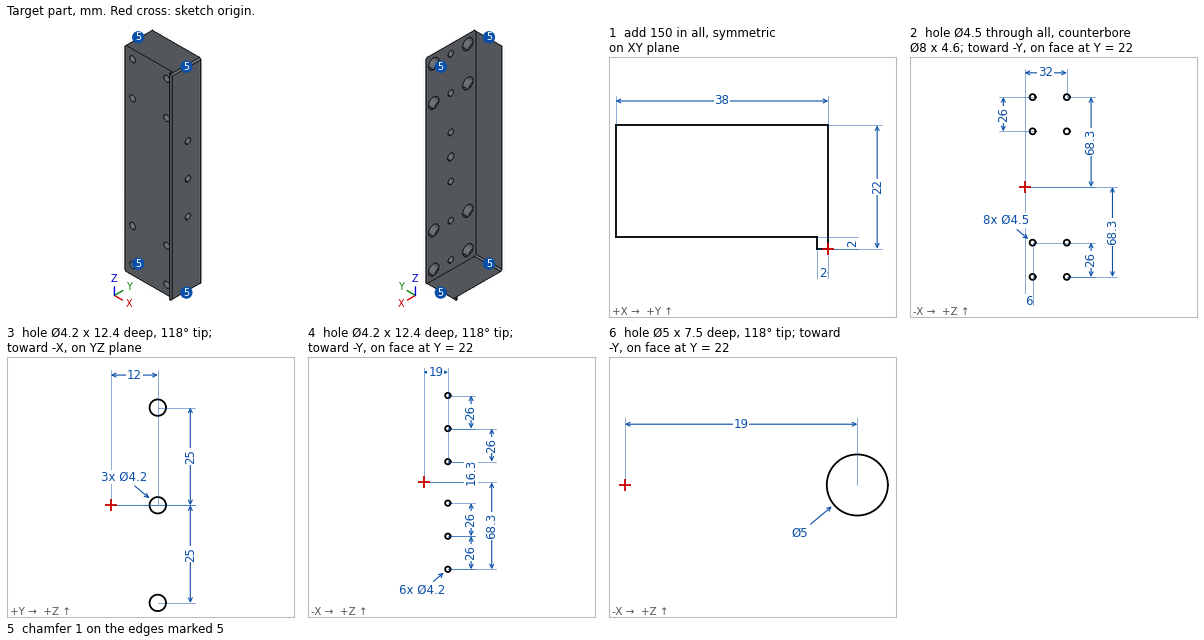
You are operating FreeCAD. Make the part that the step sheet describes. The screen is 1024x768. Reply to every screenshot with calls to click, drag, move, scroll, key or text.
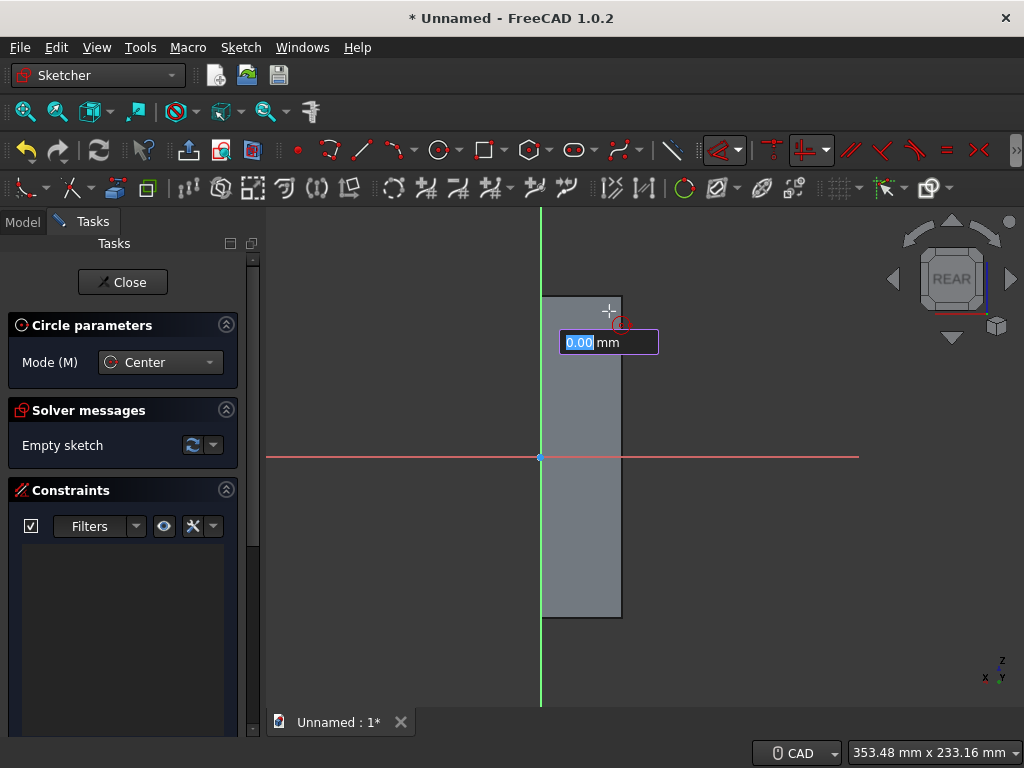
scroll(613, 307, up, 6)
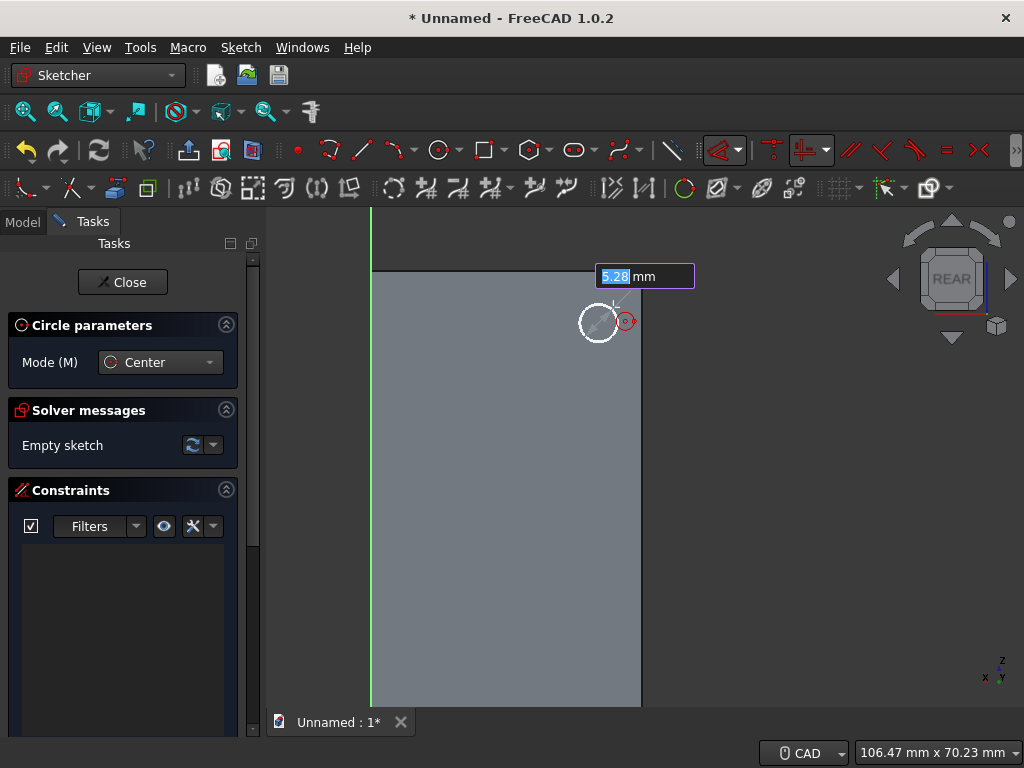
click(610, 307)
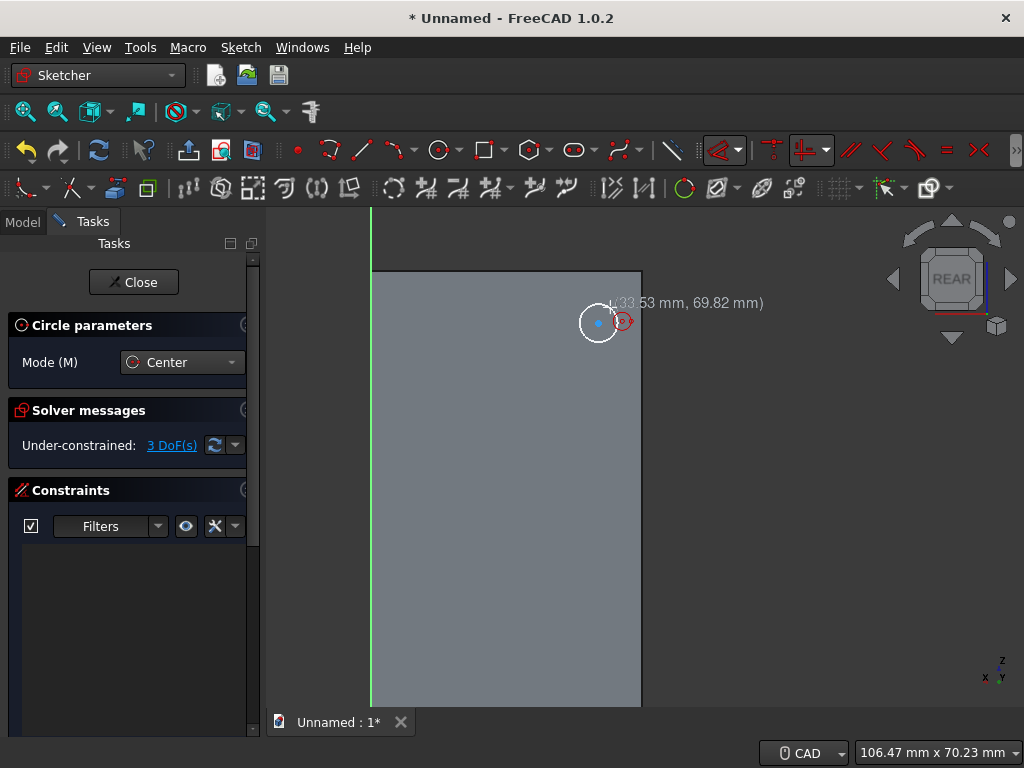
scroll(612, 307, down, 6)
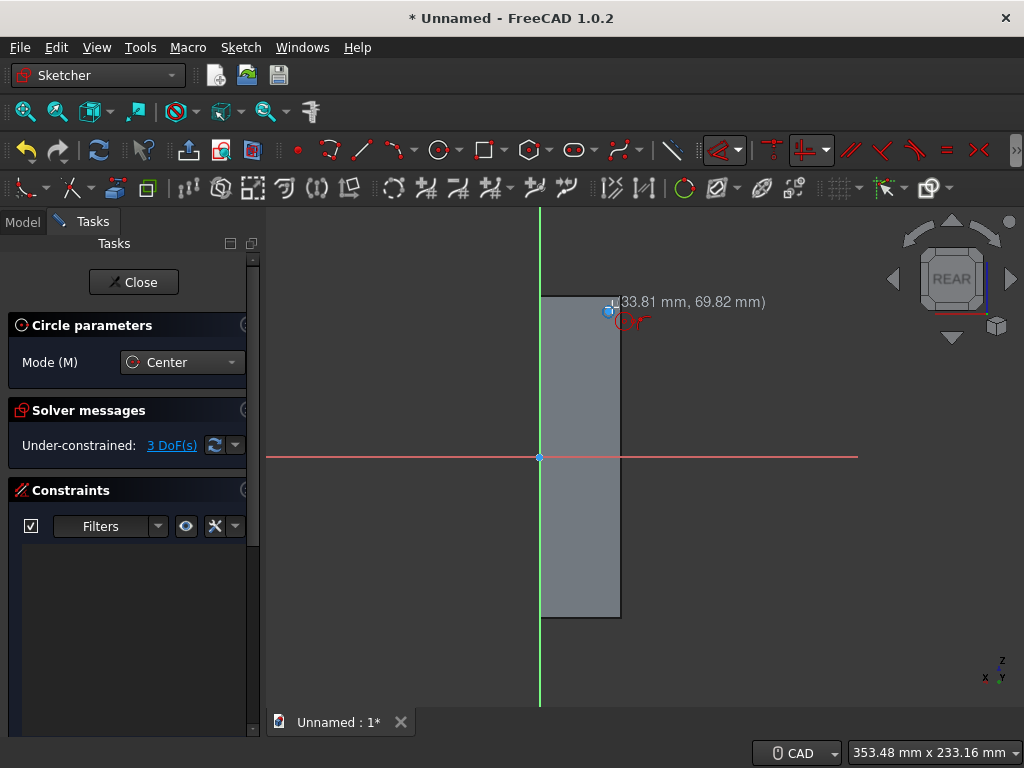
scroll(608, 604, up, 8)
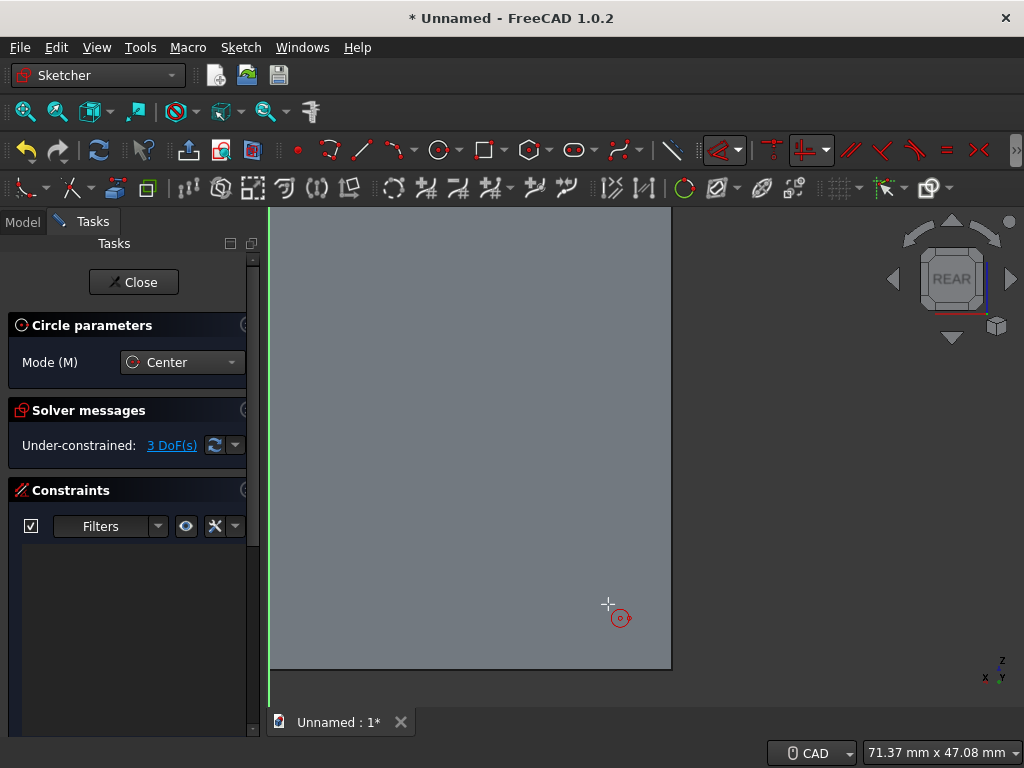
scroll(608, 605, down, 8)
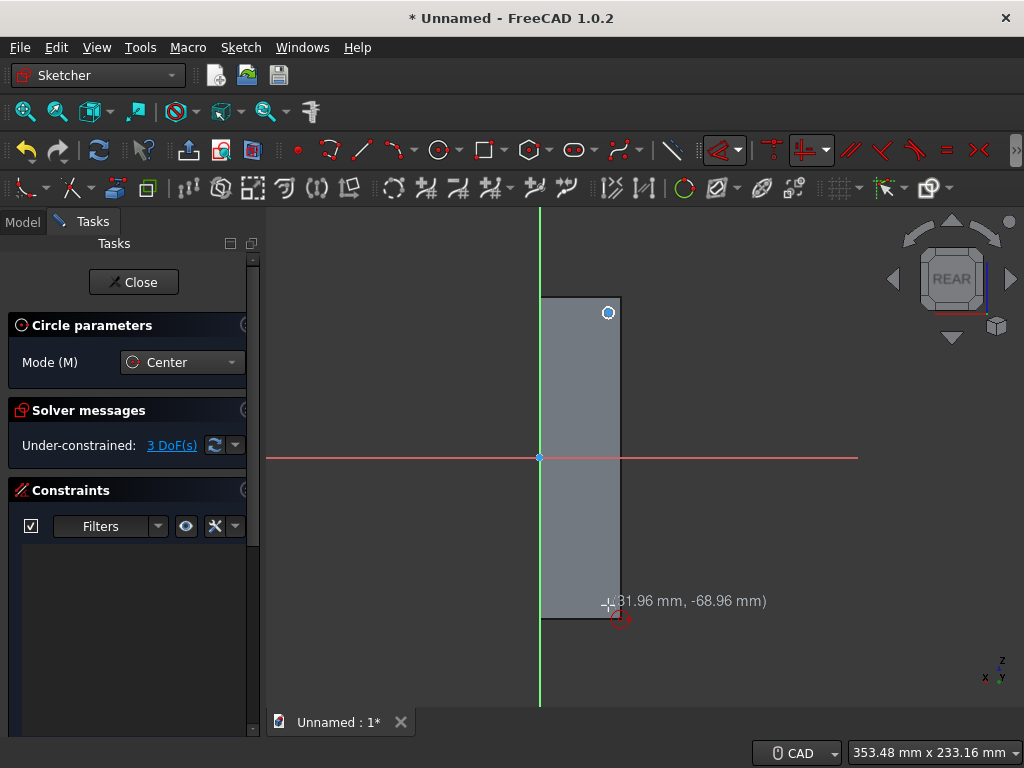
click(608, 604)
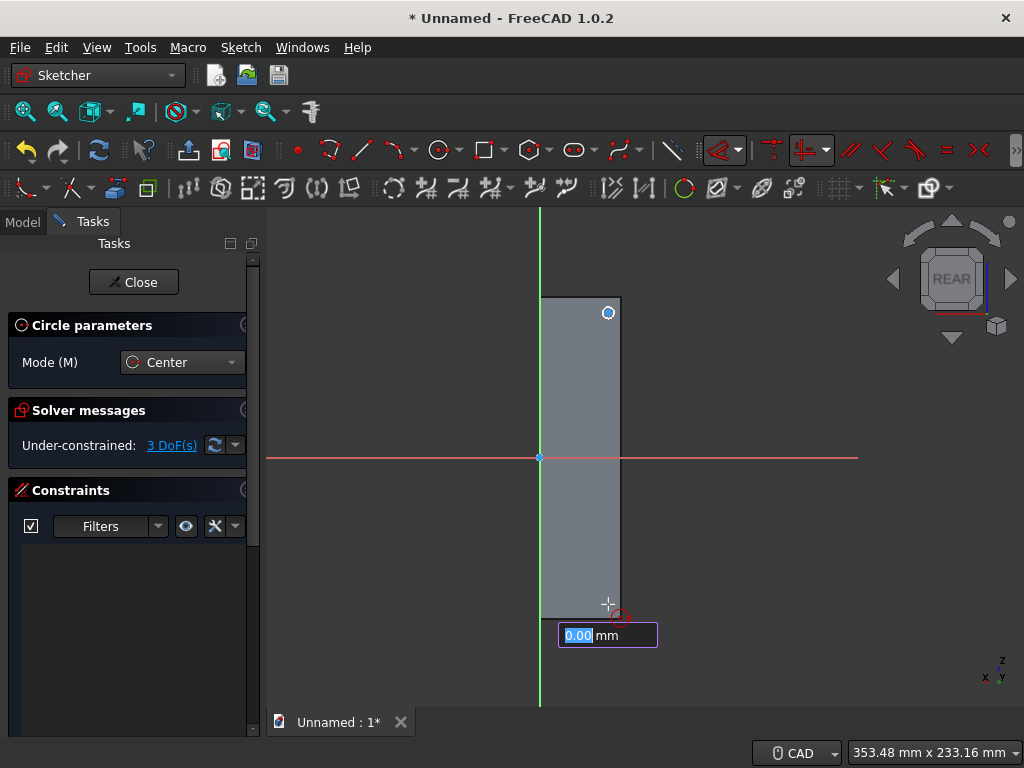
scroll(612, 601, up, 6)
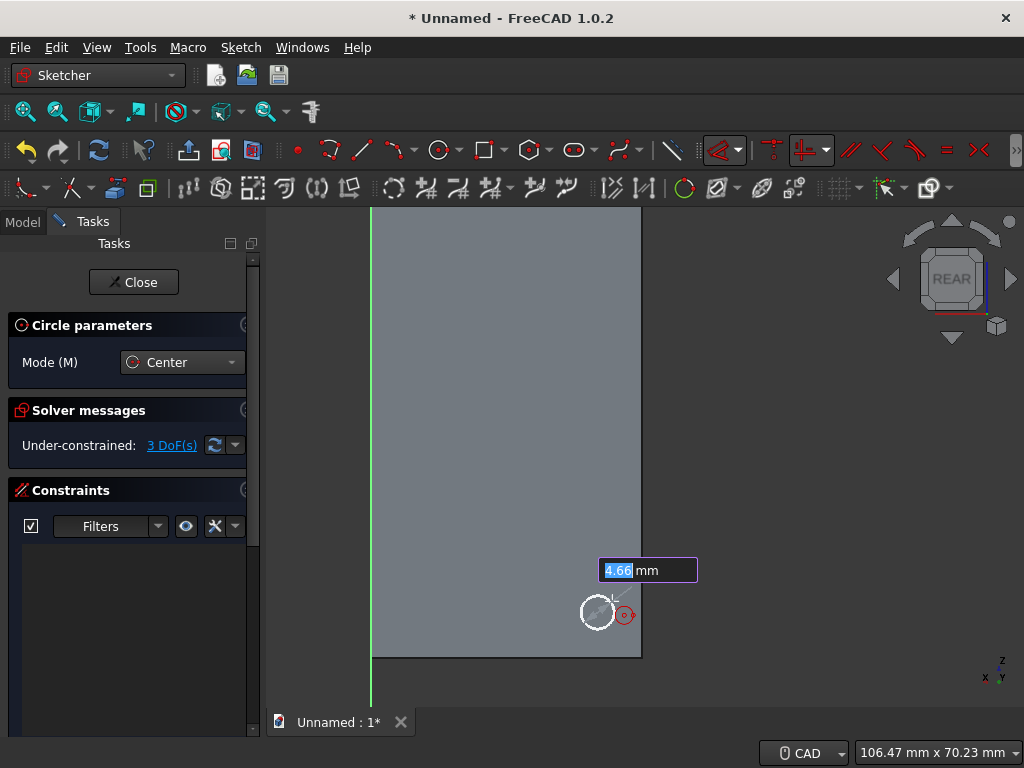
click(610, 599)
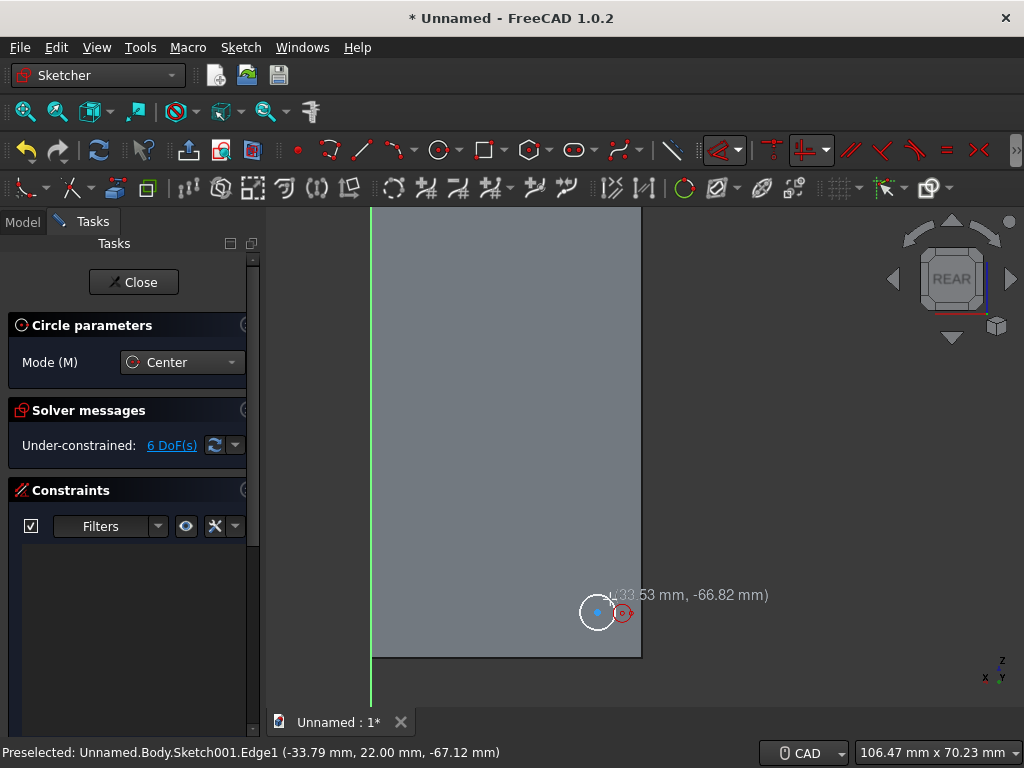
scroll(414, 425, up, 2)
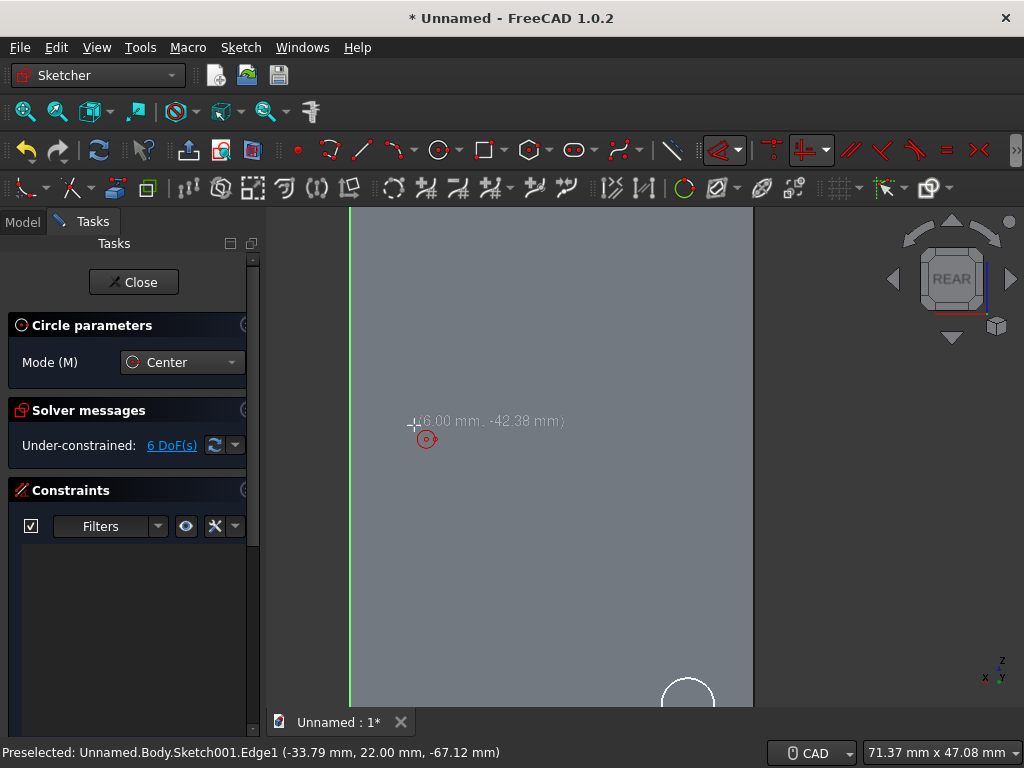
scroll(588, 579, down, 8)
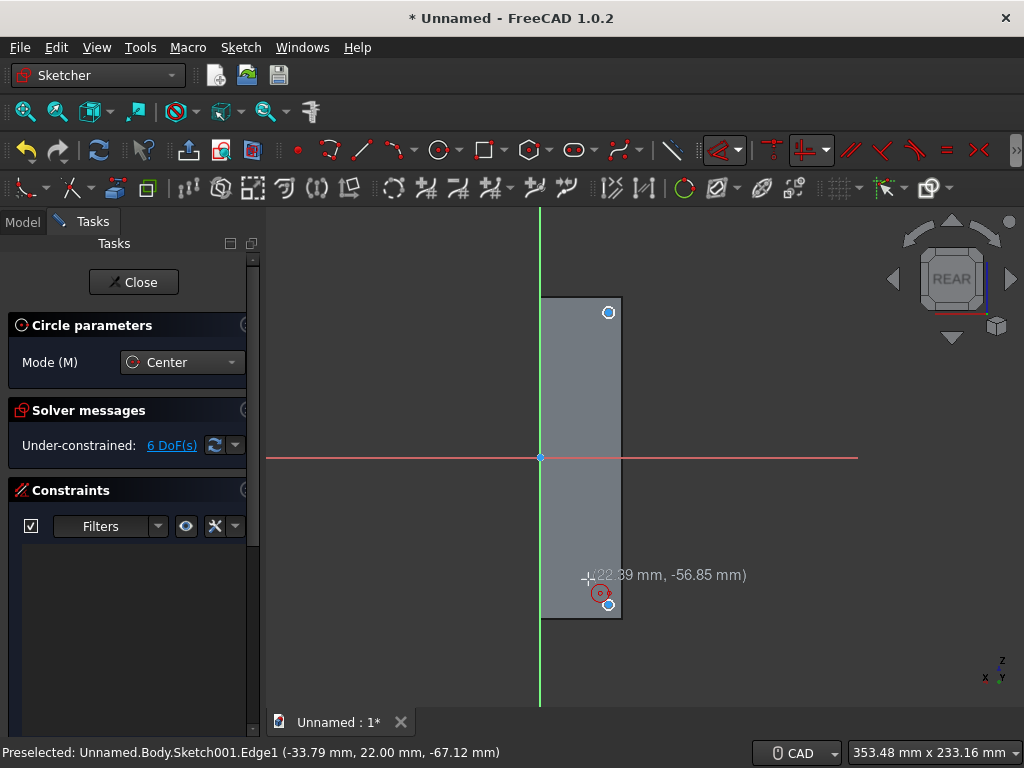
scroll(553, 549, up, 2)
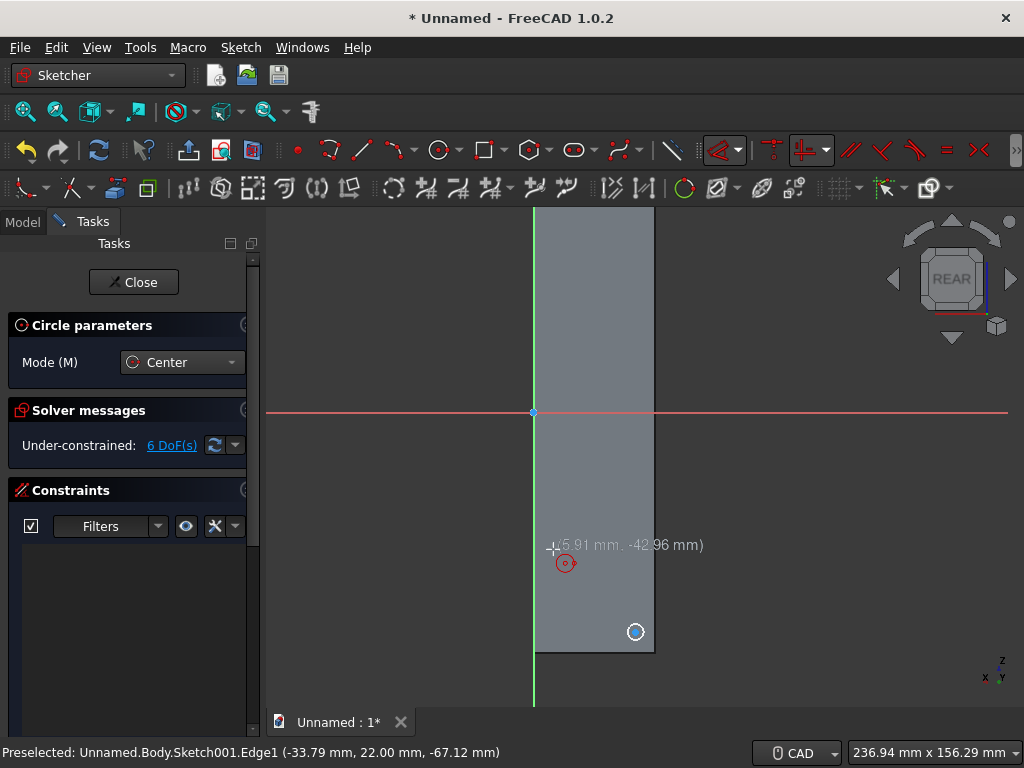
click(553, 548)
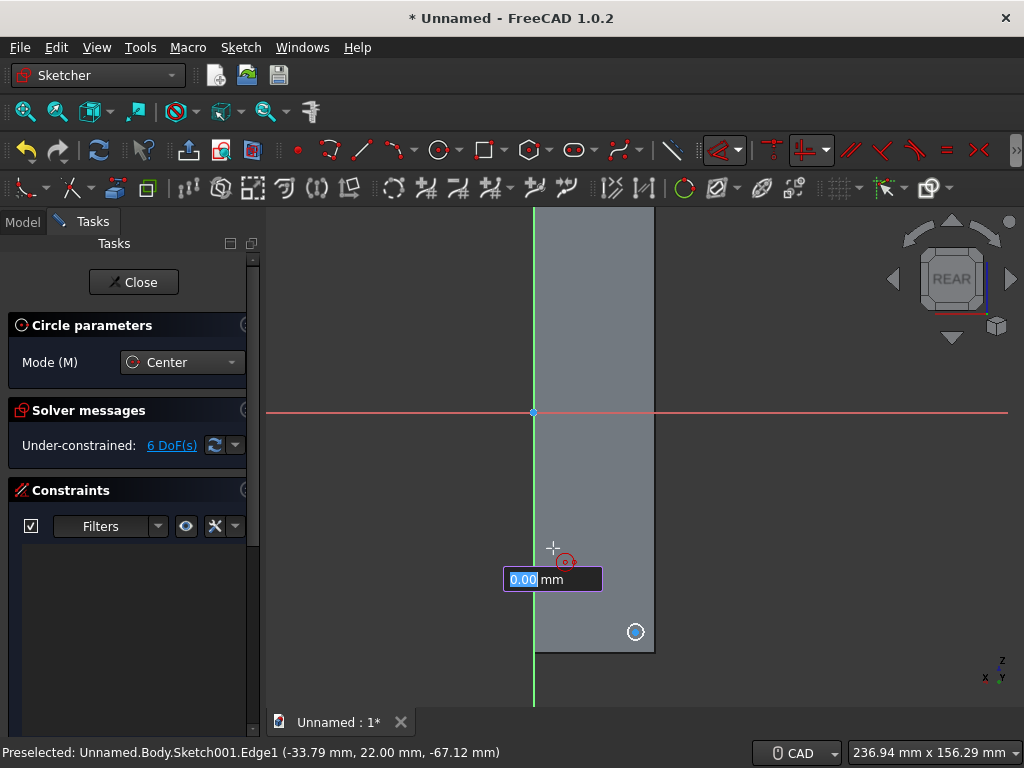
scroll(558, 543, up, 4)